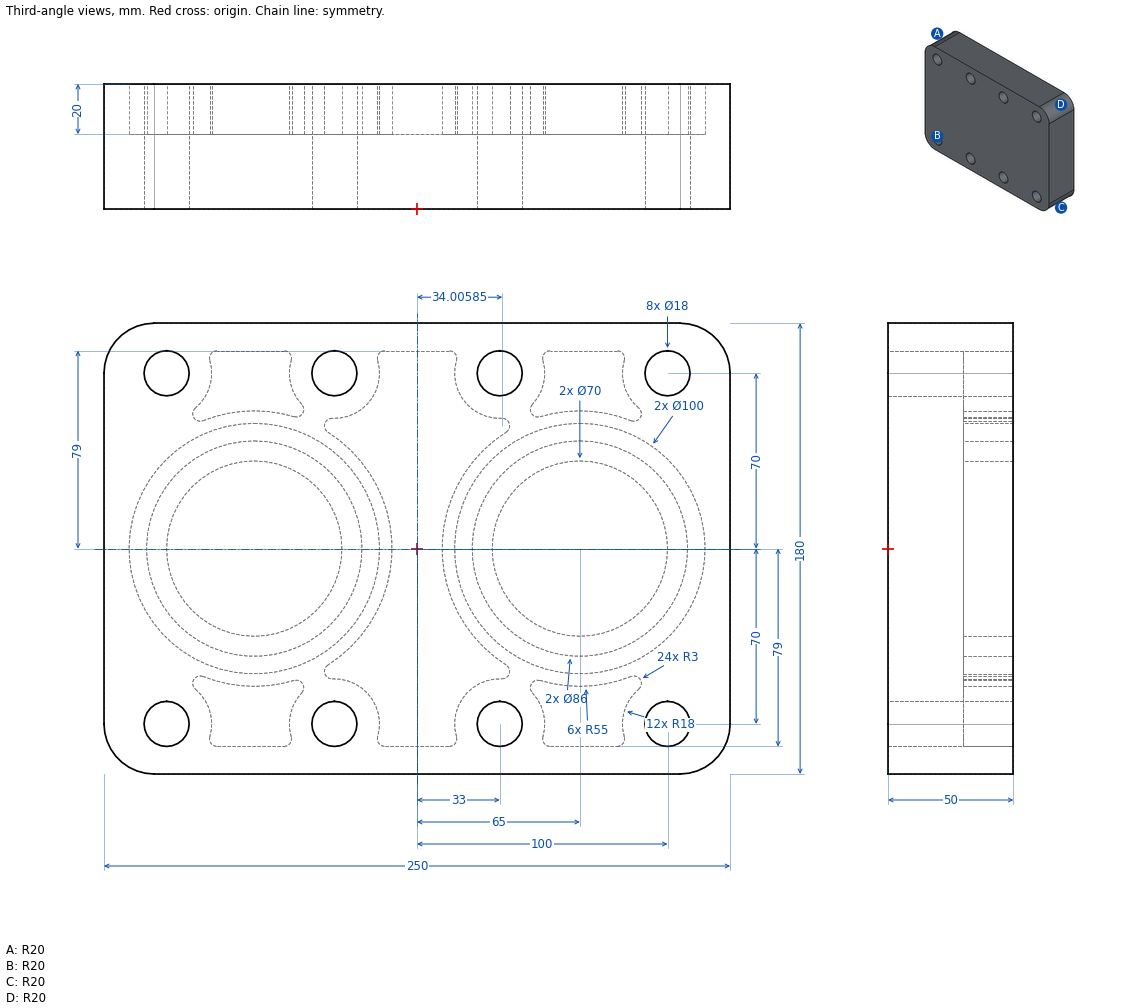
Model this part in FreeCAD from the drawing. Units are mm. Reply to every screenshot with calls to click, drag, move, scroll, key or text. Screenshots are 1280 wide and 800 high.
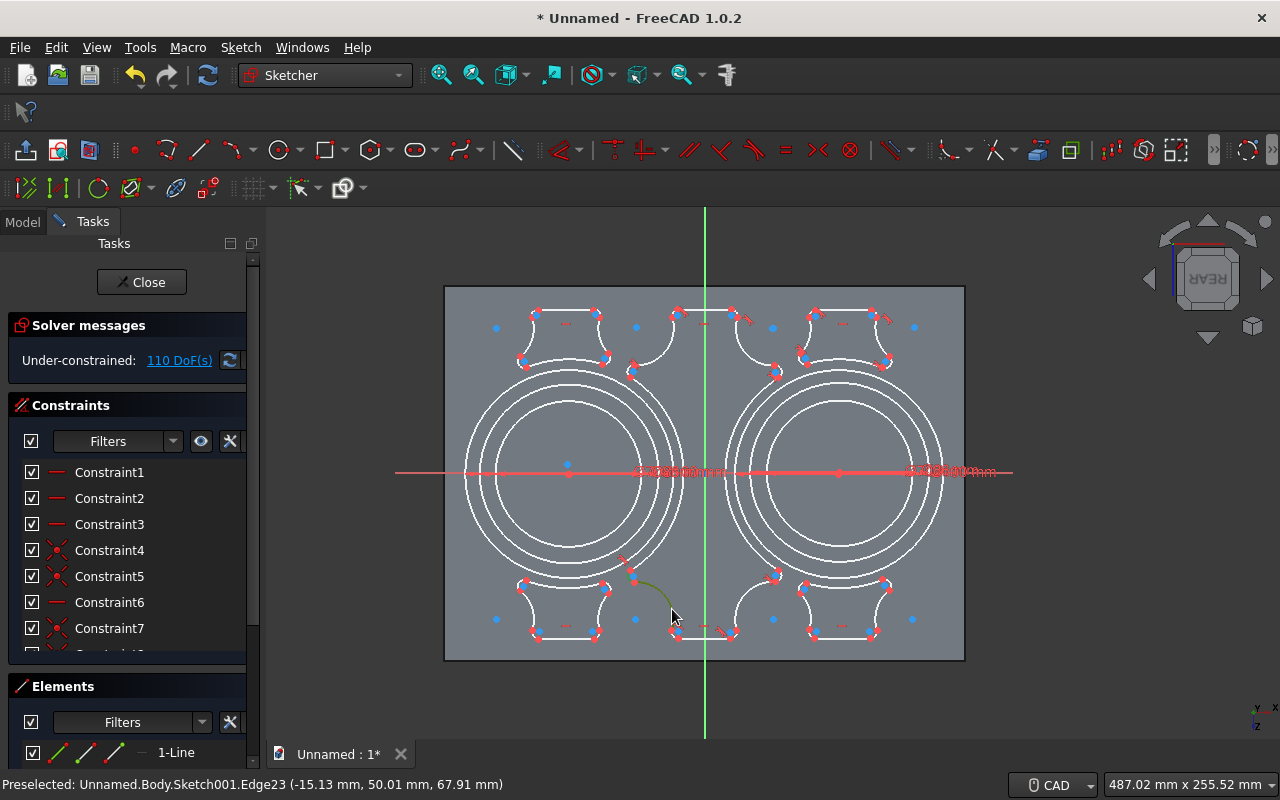
click(754, 150)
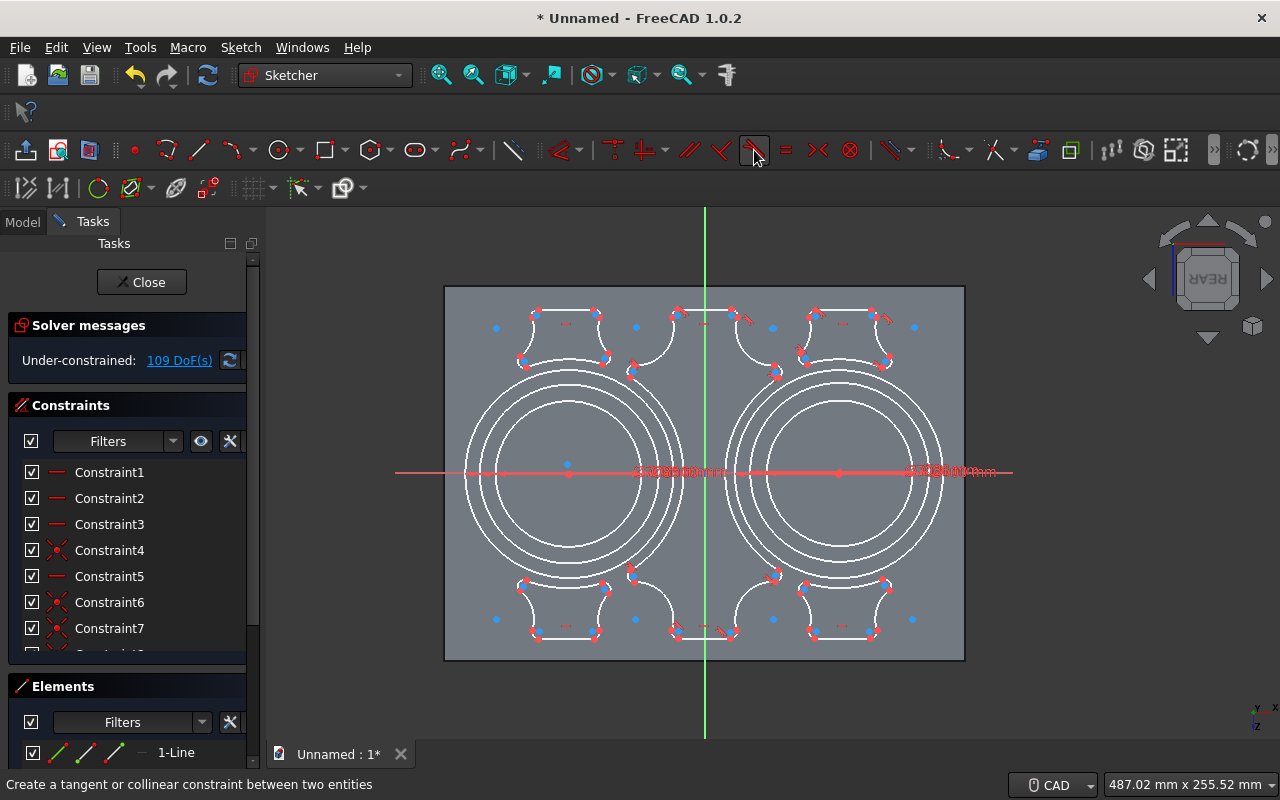
click(672, 609)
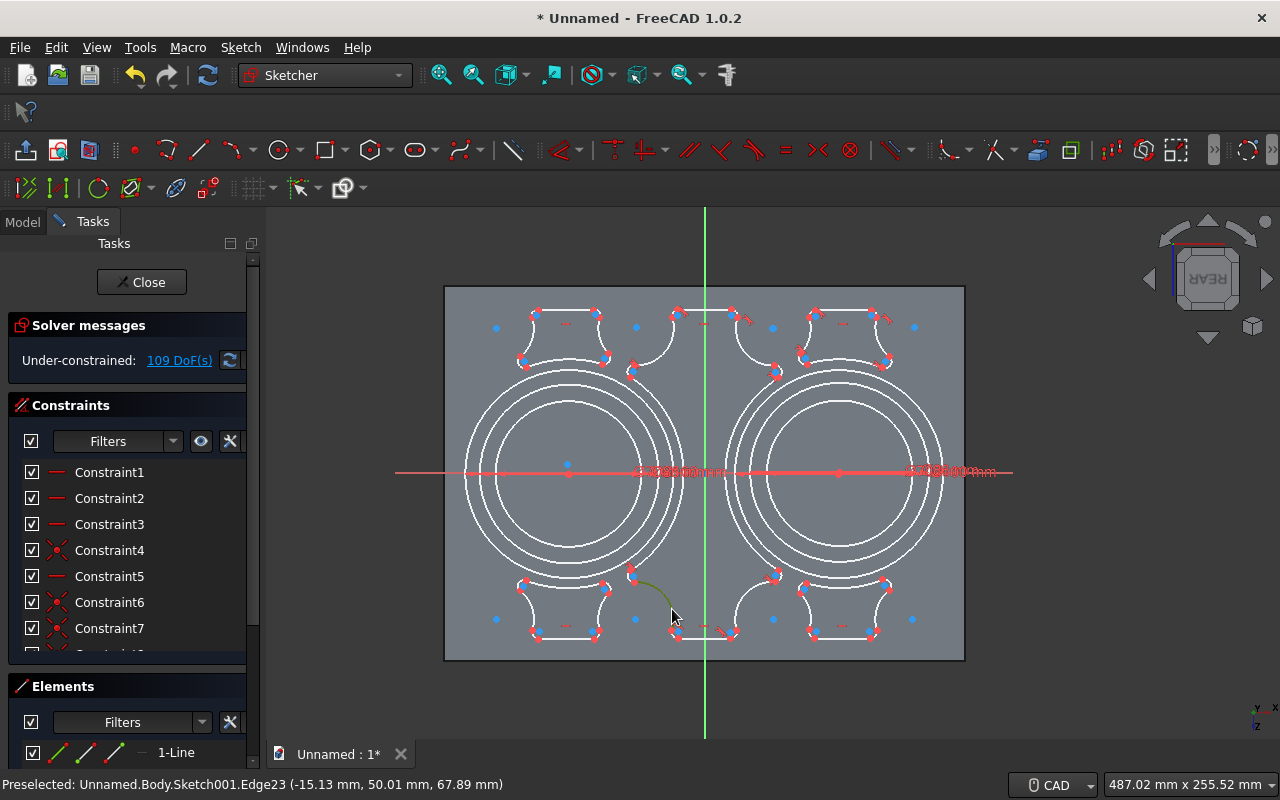
scroll(673, 636, up, 5)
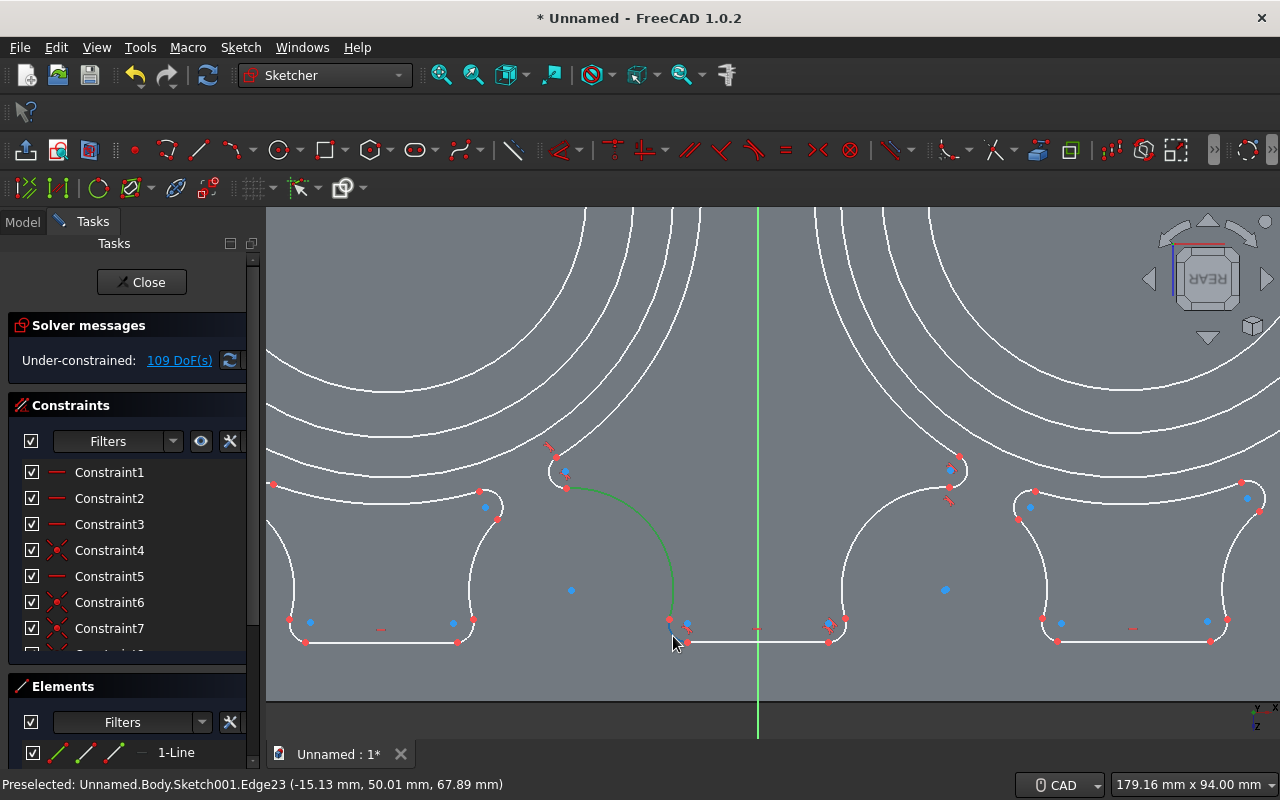
click(673, 635)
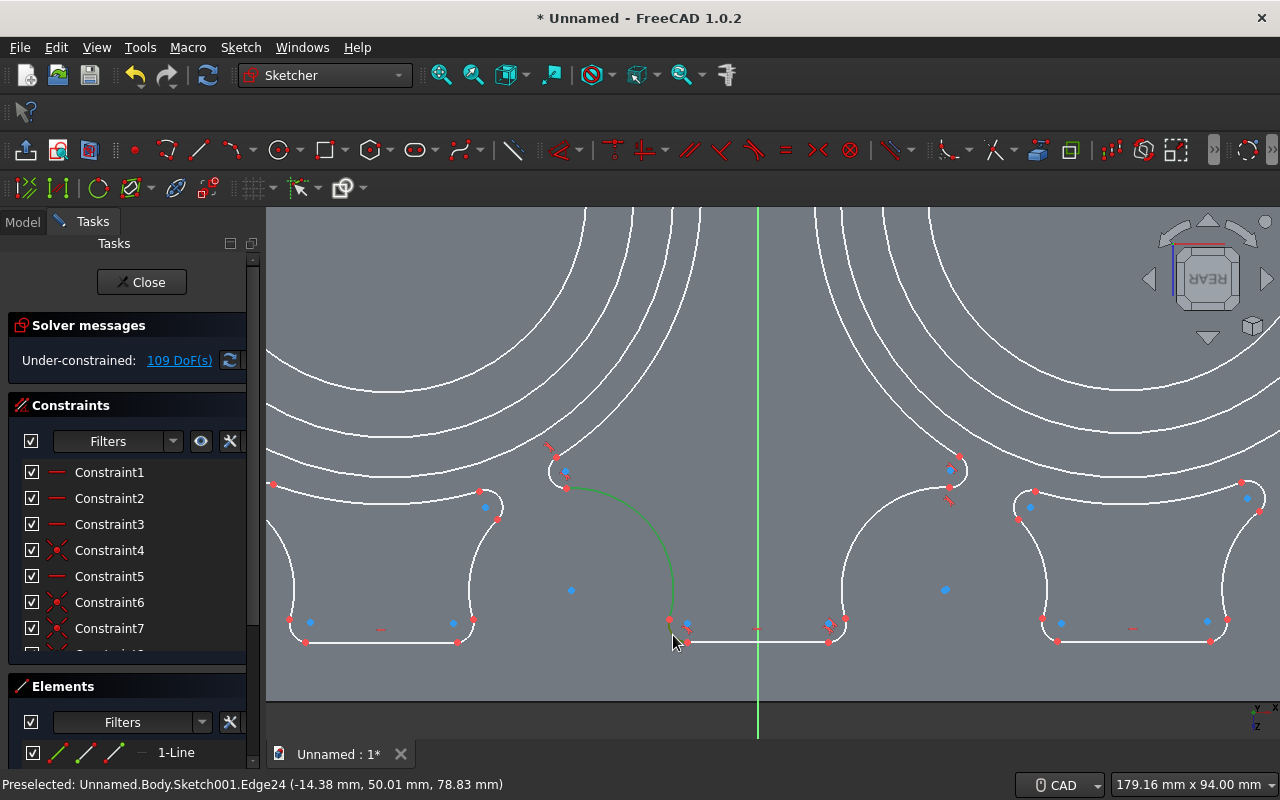
click(754, 150)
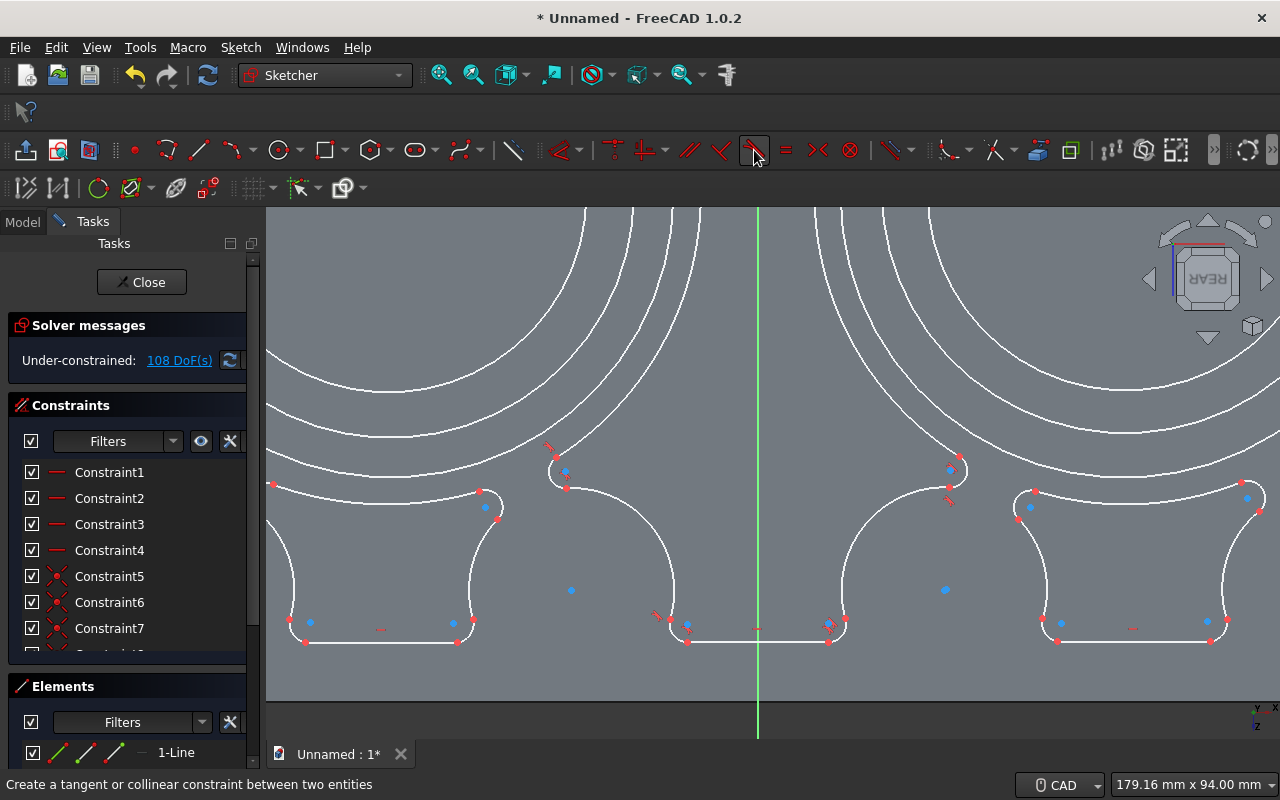
scroll(673, 636, down, 5)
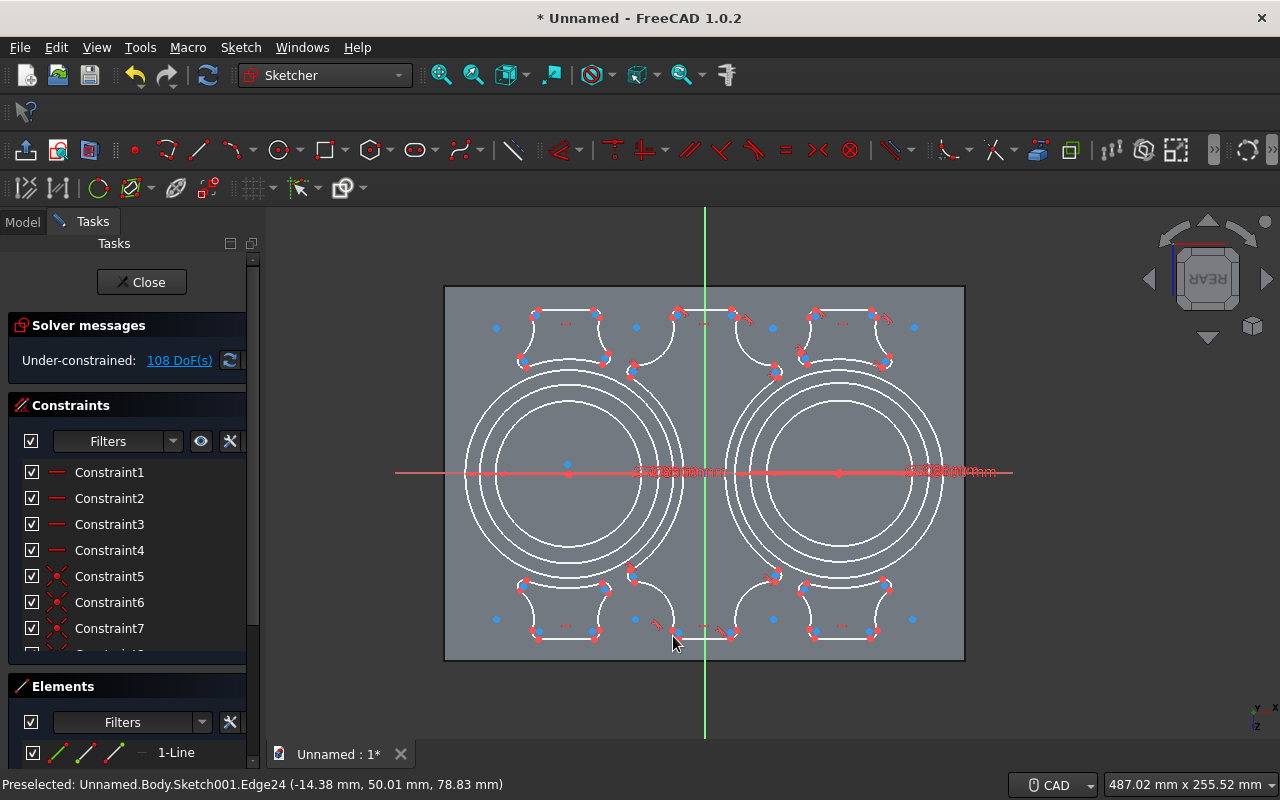
click(577, 310)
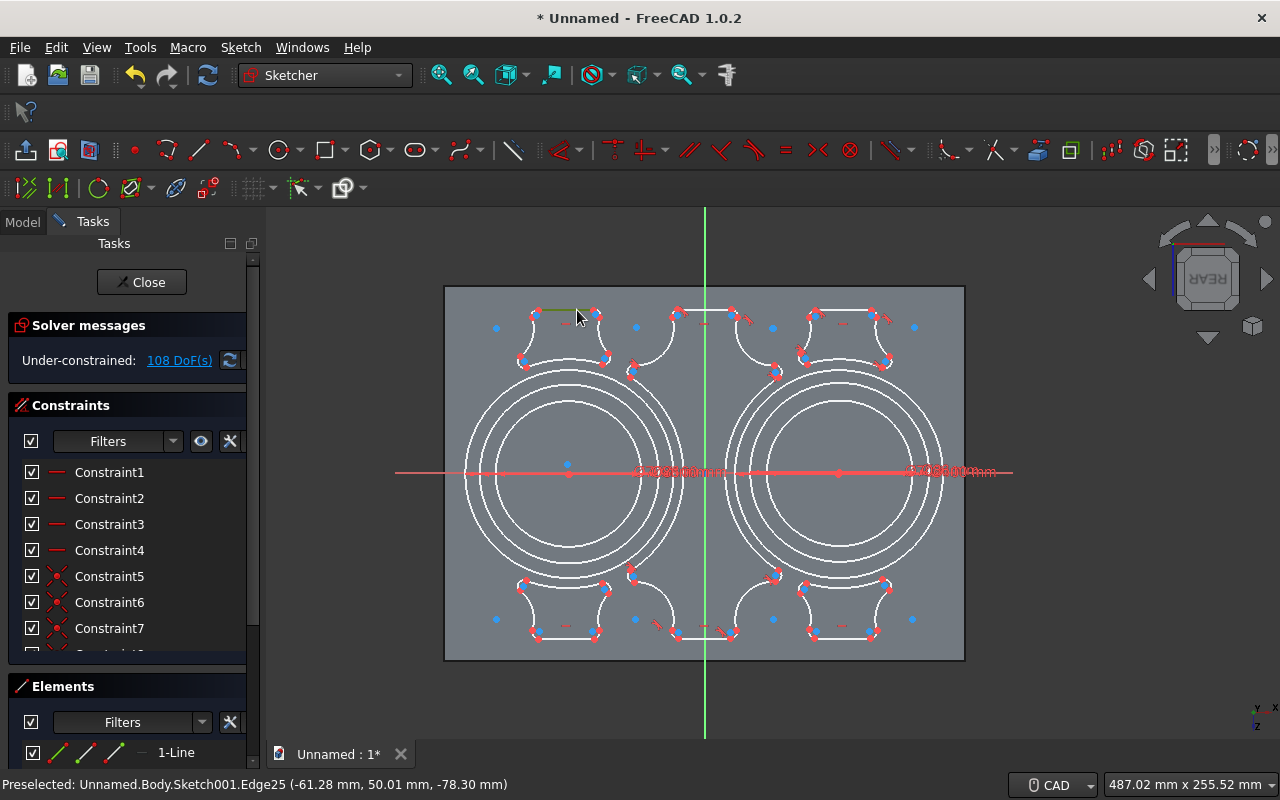
scroll(533, 312, up, 5)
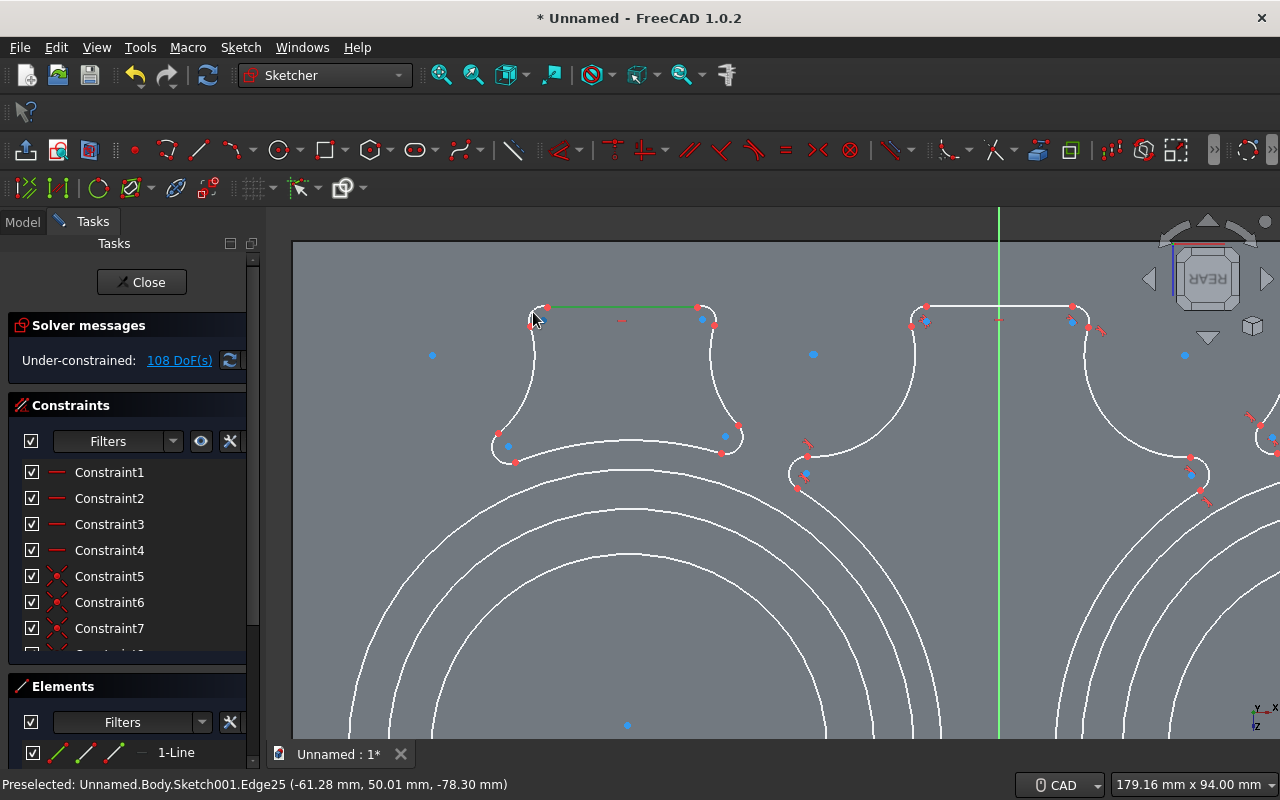
click(533, 311)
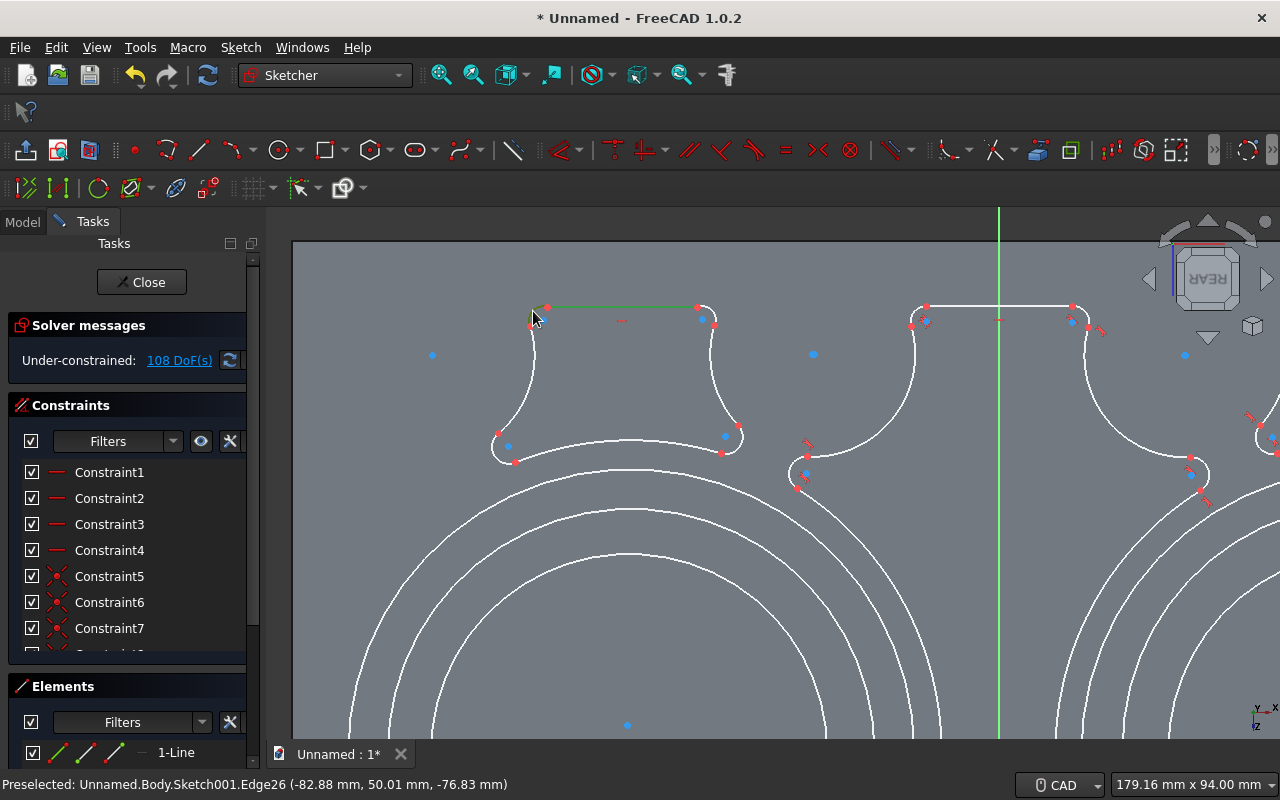
click(754, 150)